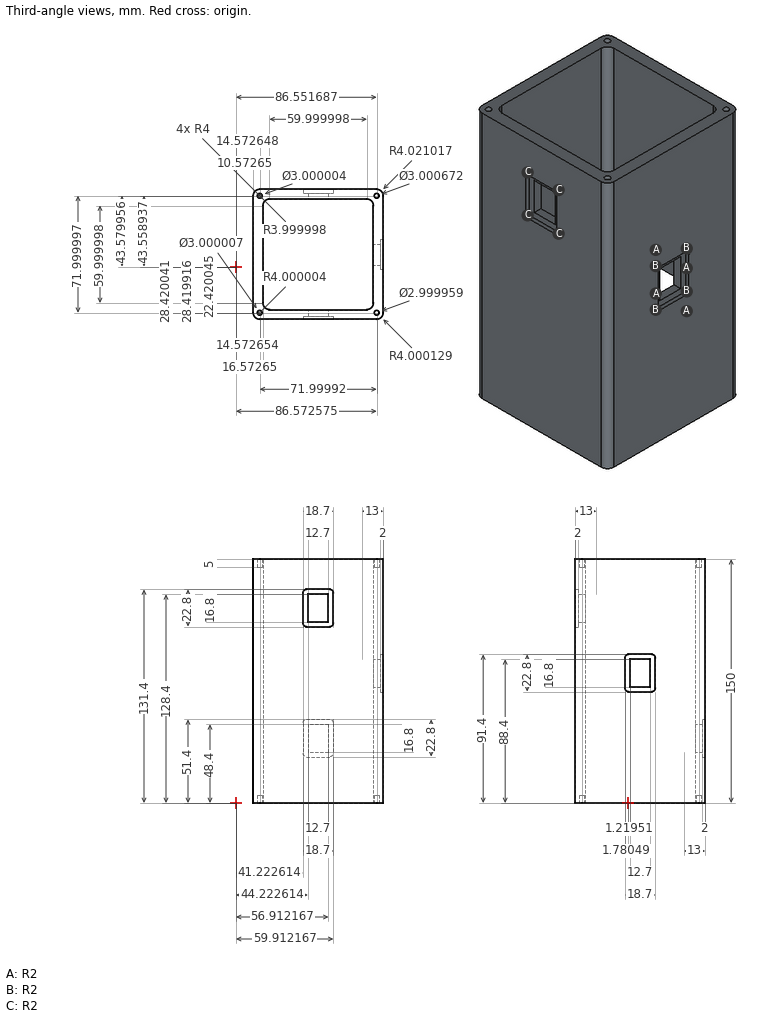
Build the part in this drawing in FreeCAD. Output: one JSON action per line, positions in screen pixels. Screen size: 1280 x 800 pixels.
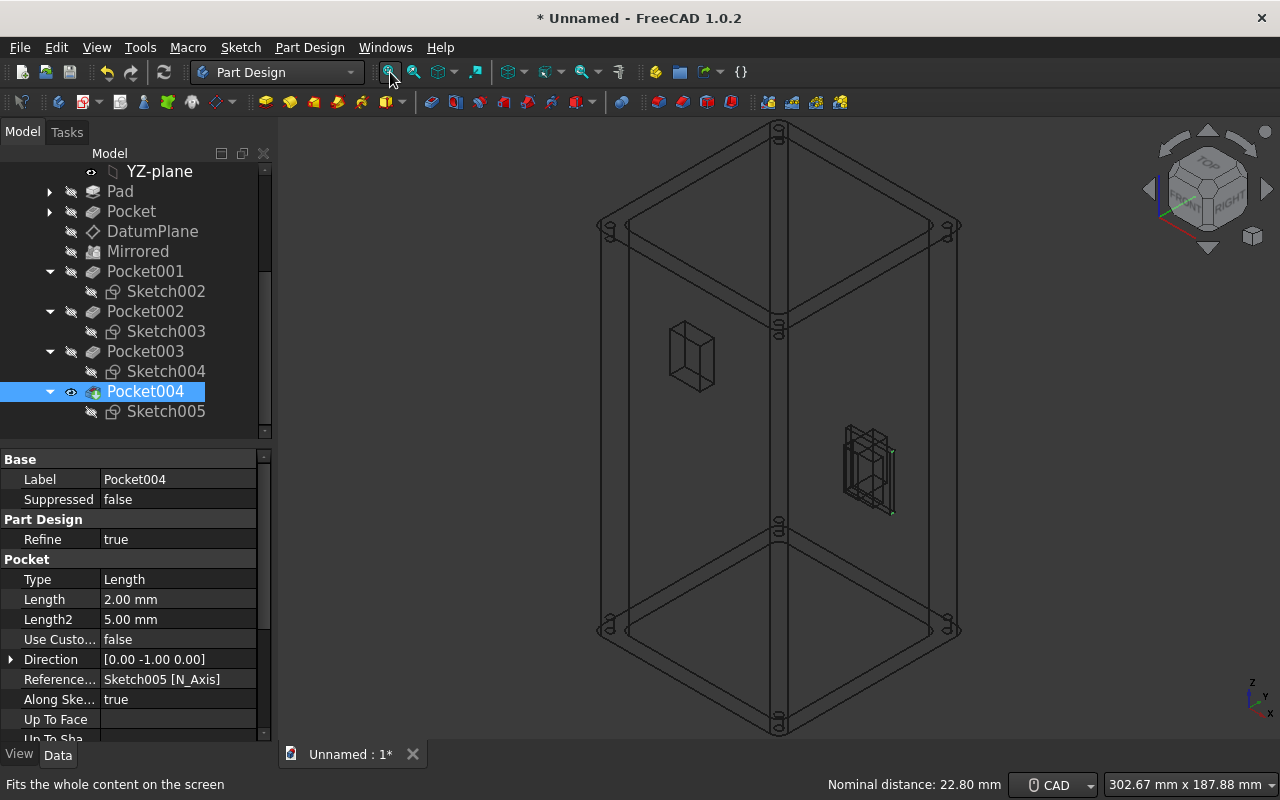
{"action": "key", "text": "2"}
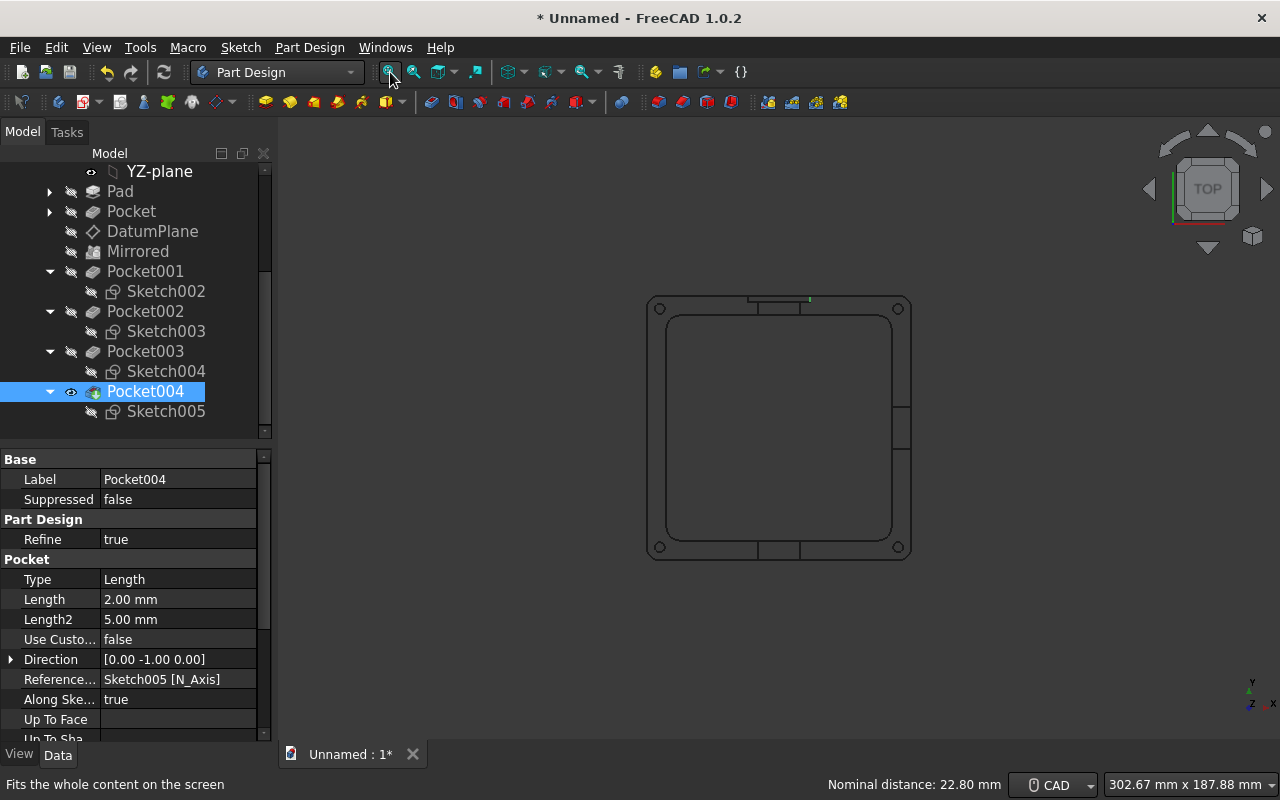
{"action": "left_click", "coordinate": [390, 72]}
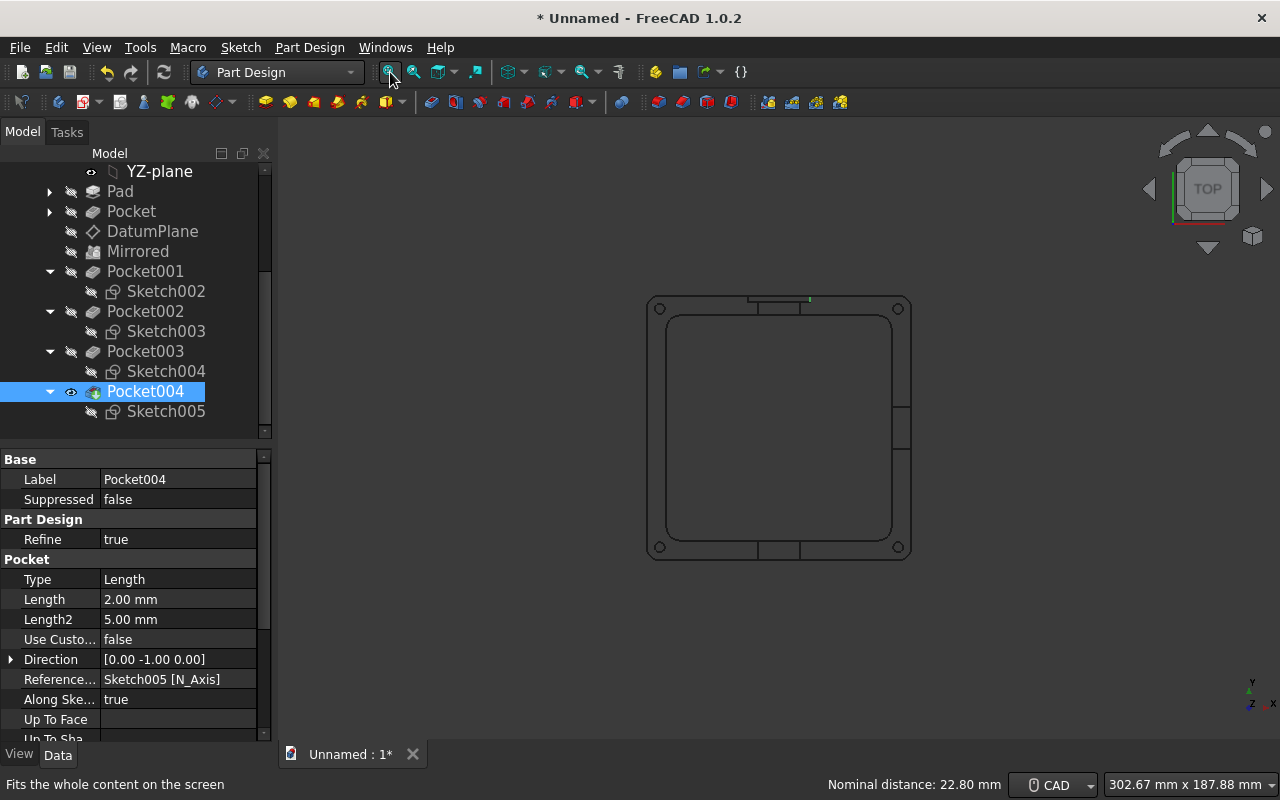
{"action": "scroll", "coordinate": [748, 298], "scroll_direction": "up", "scroll_amount": 9}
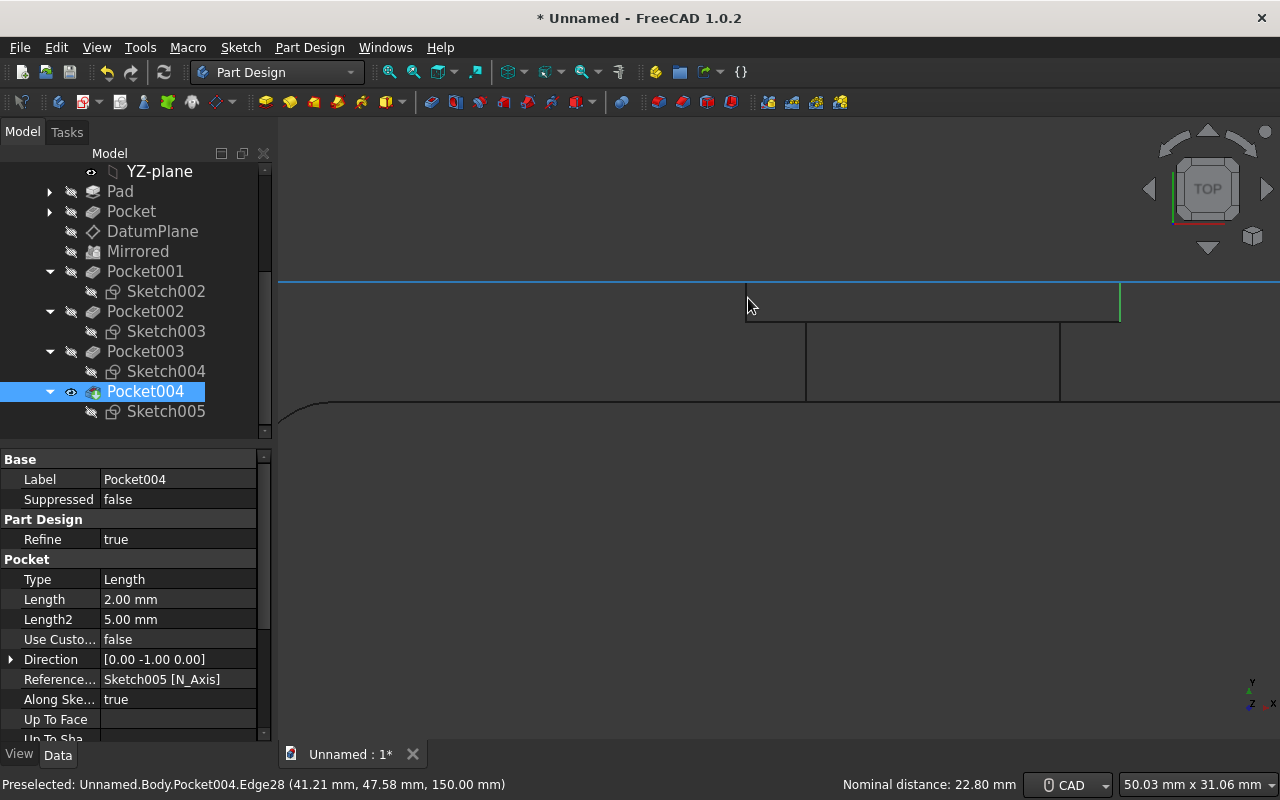
{"action": "left_click", "coordinate": [746, 301], "text": "ctrl"}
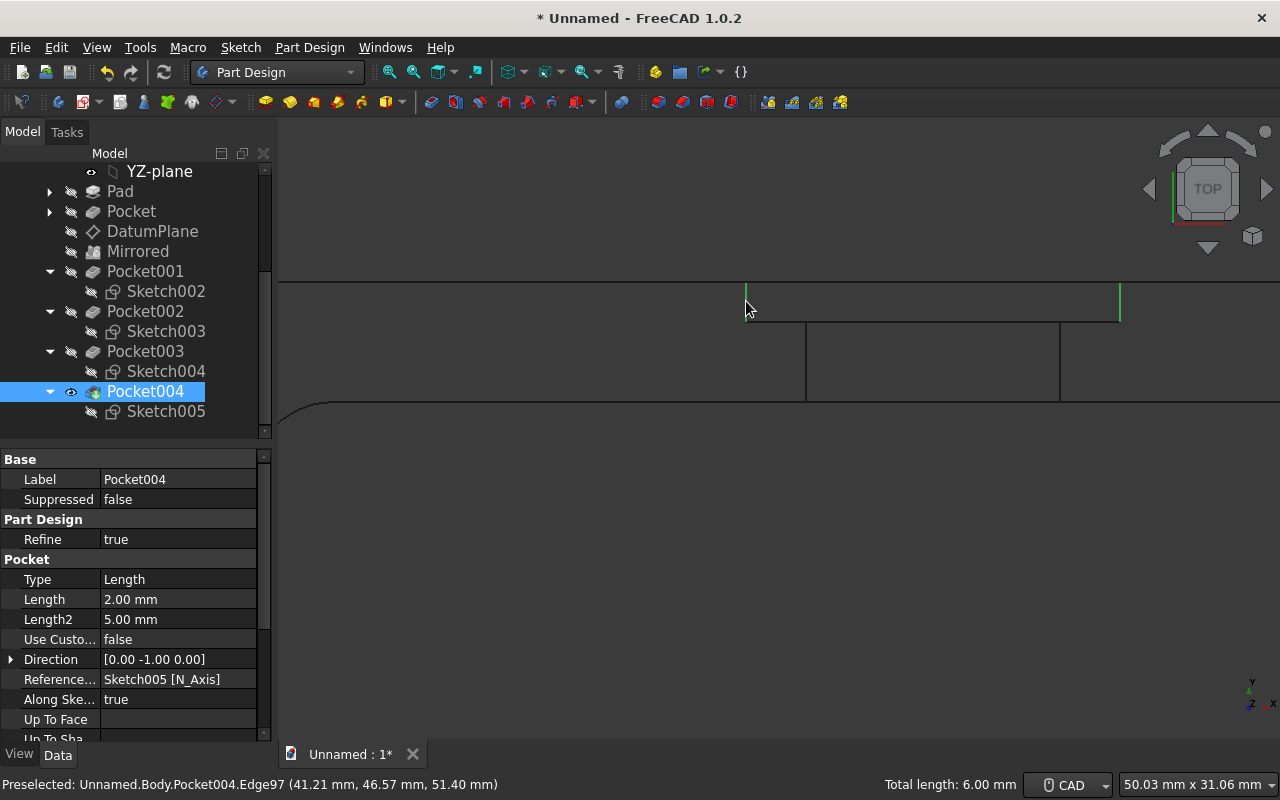
{"action": "left_click", "coordinate": [390, 72]}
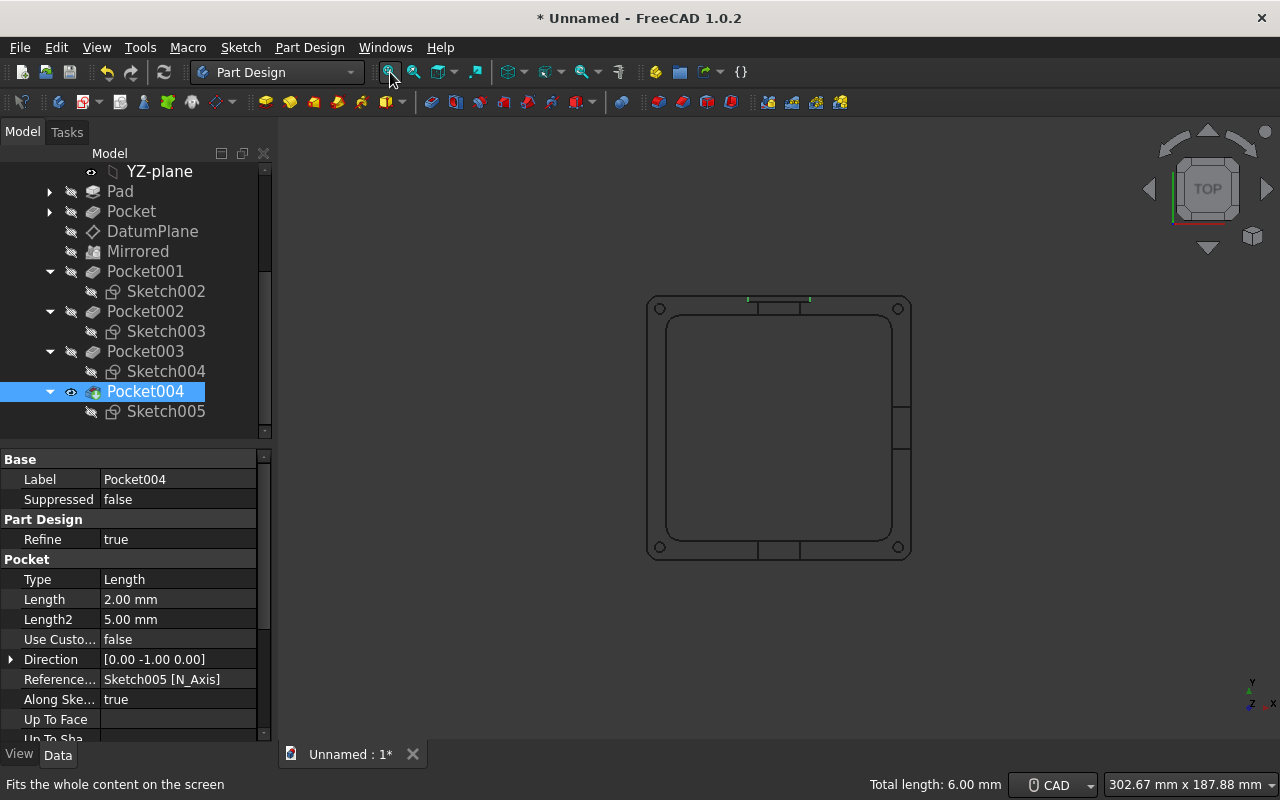
{"action": "key", "text": "1"}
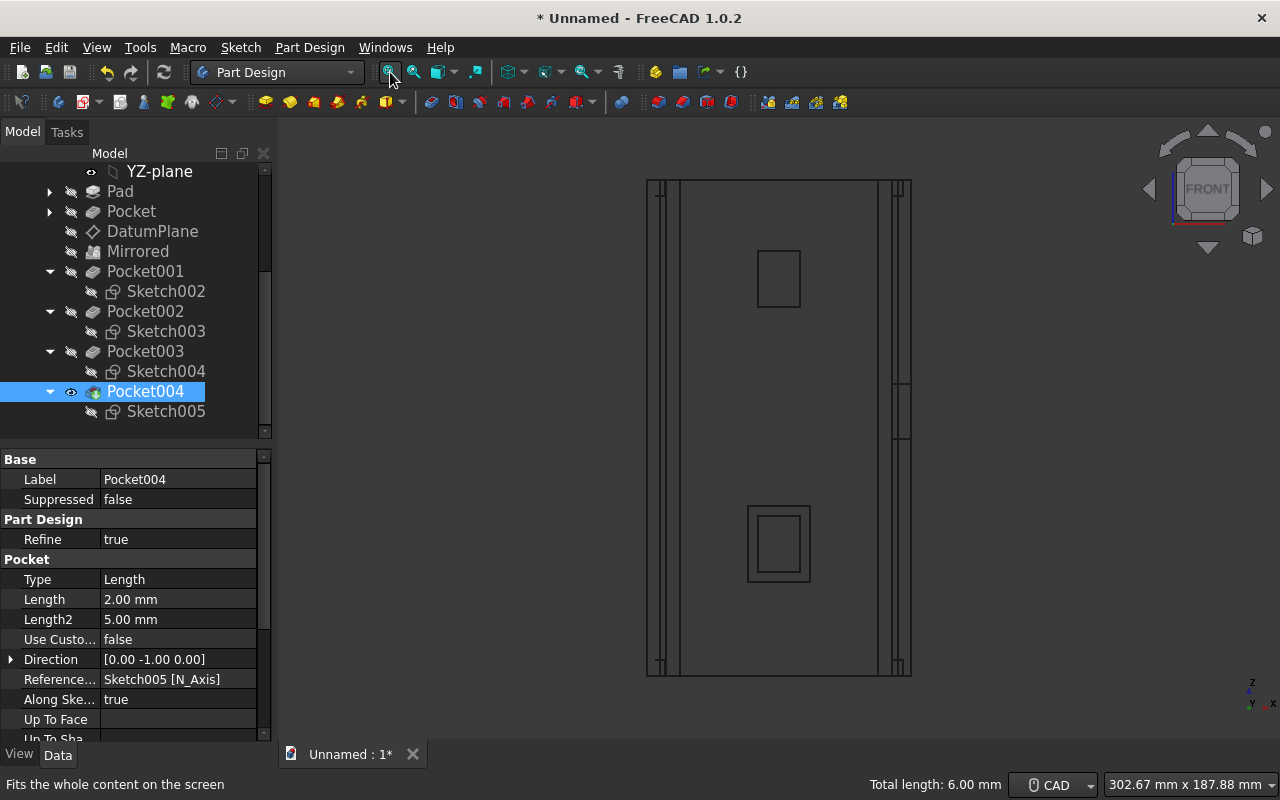
{"action": "scroll", "coordinate": [748, 581], "scroll_direction": "up", "scroll_amount": 9}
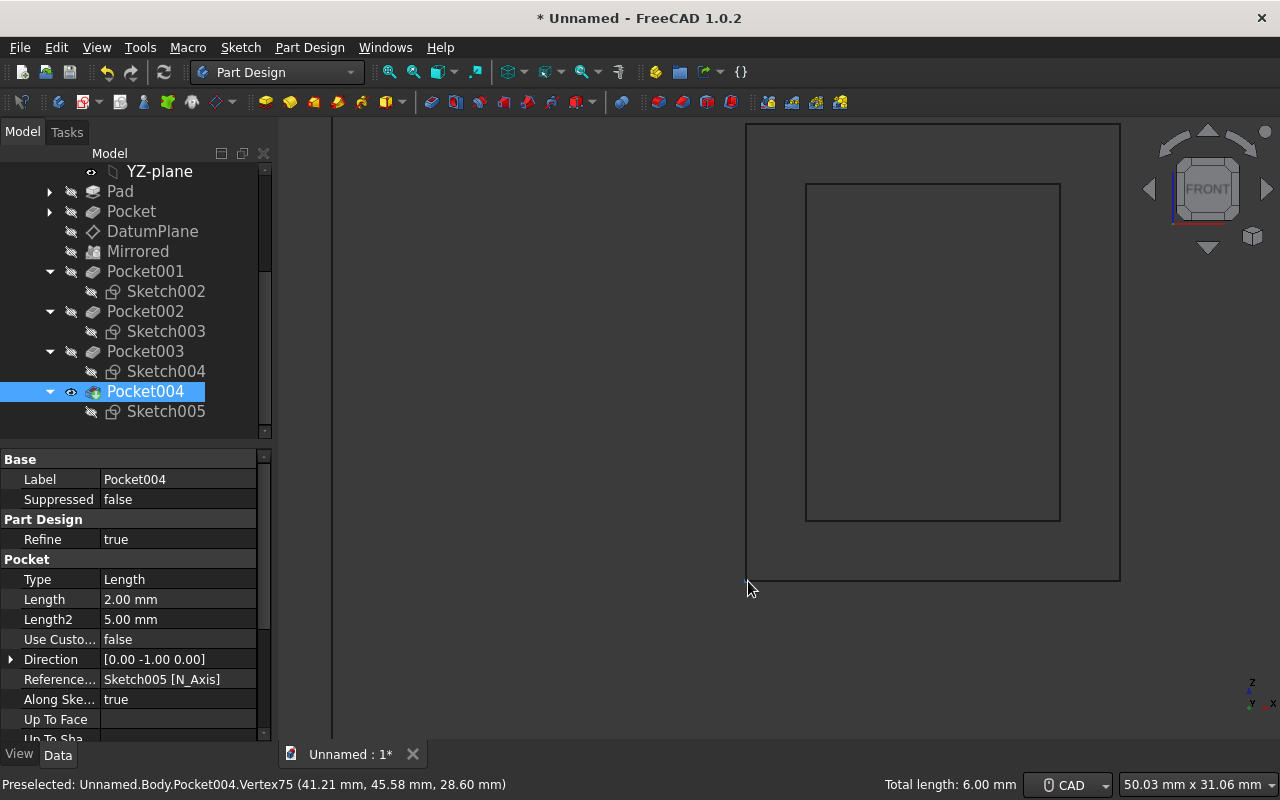
{"action": "left_click", "coordinate": [390, 72]}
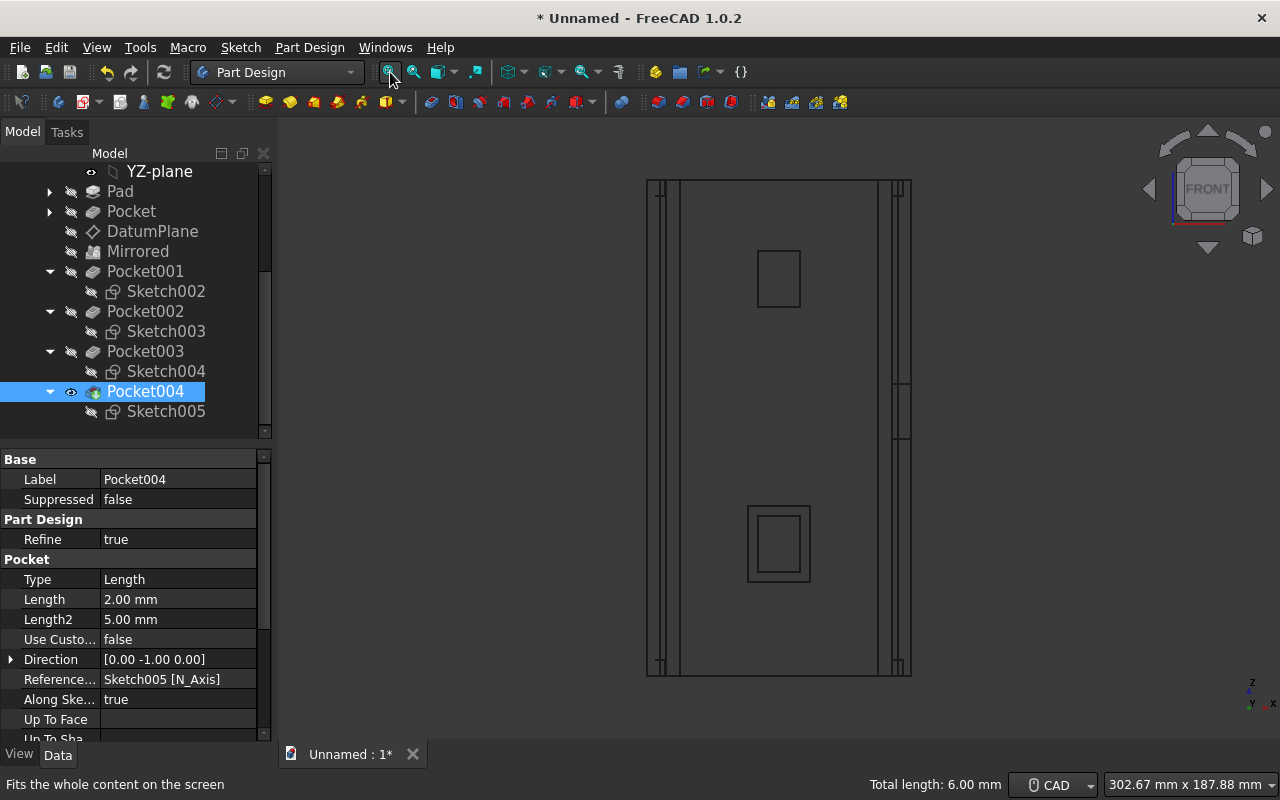
{"action": "key", "text": "3"}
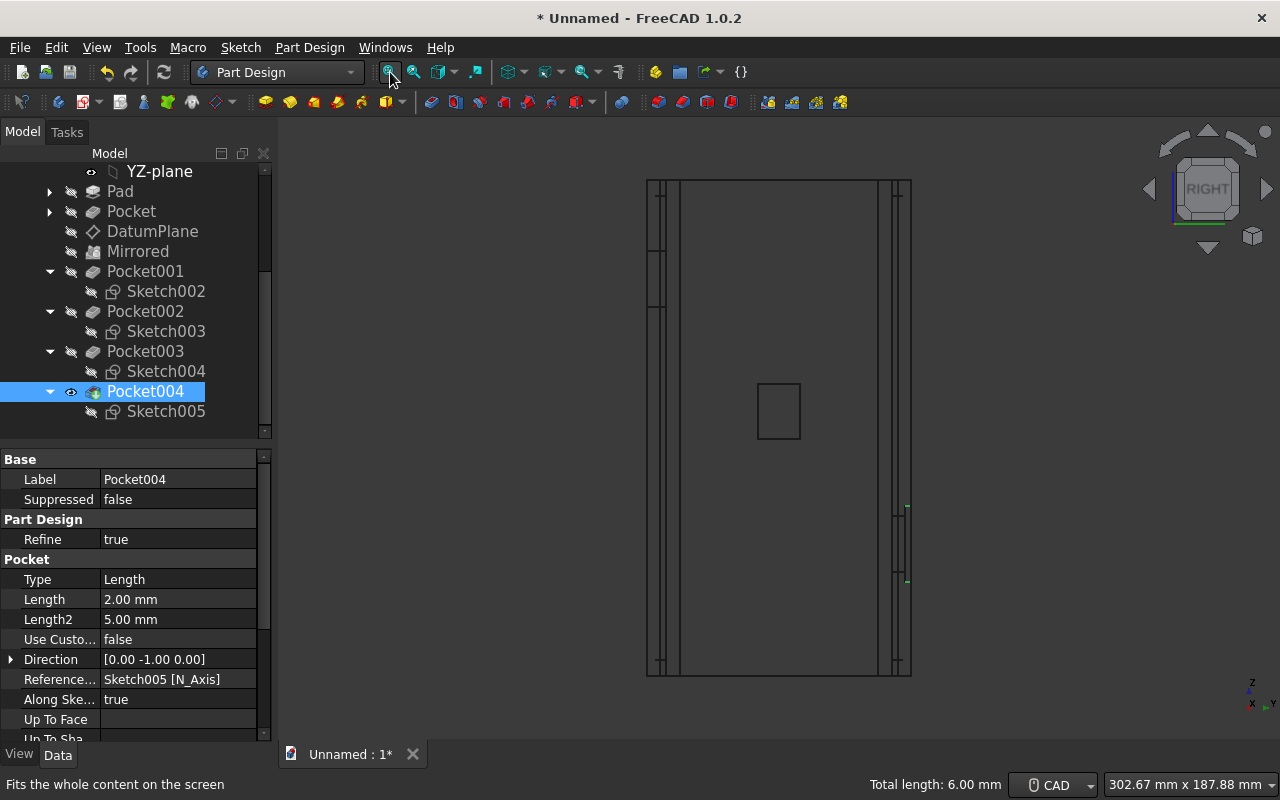
{"action": "scroll", "coordinate": [908, 581], "scroll_direction": "up", "scroll_amount": 9}